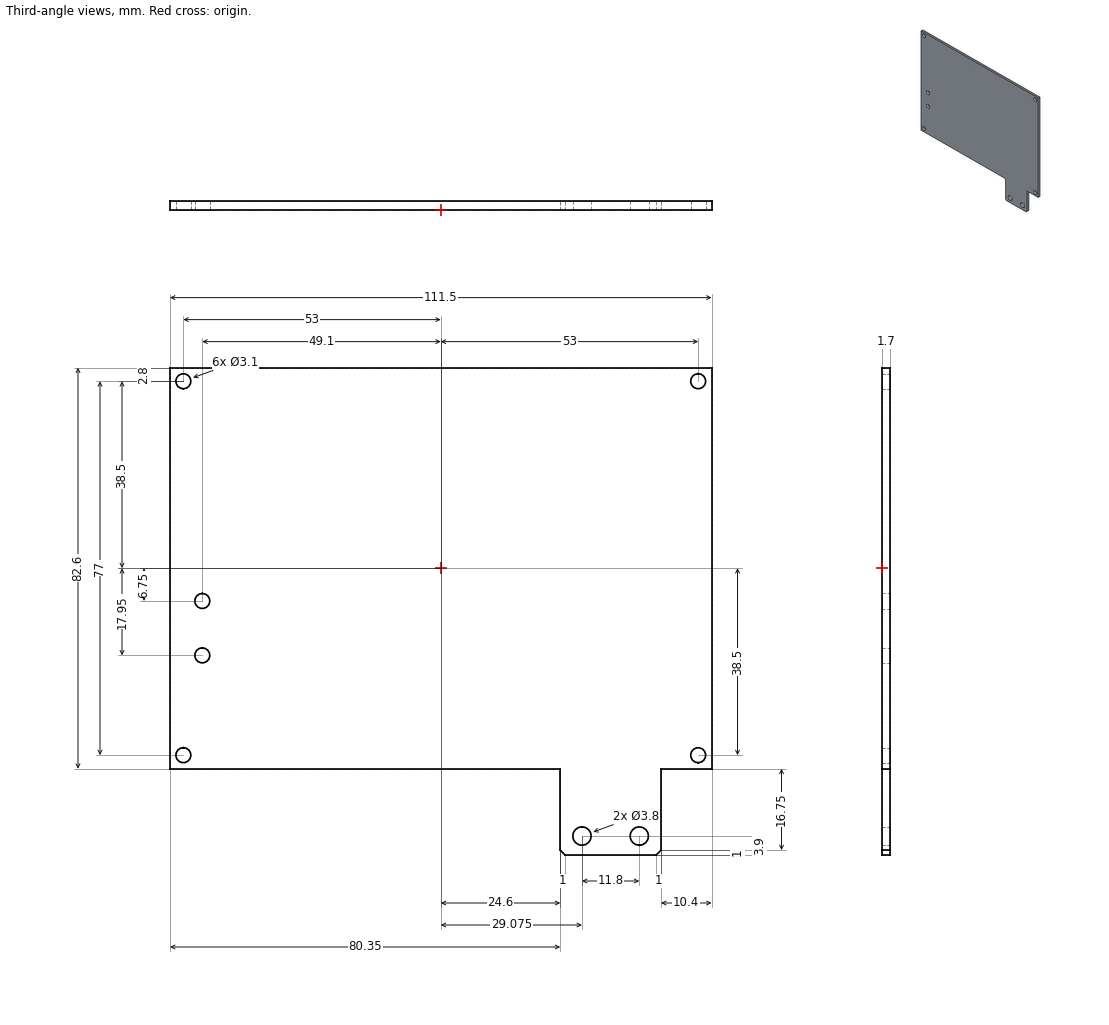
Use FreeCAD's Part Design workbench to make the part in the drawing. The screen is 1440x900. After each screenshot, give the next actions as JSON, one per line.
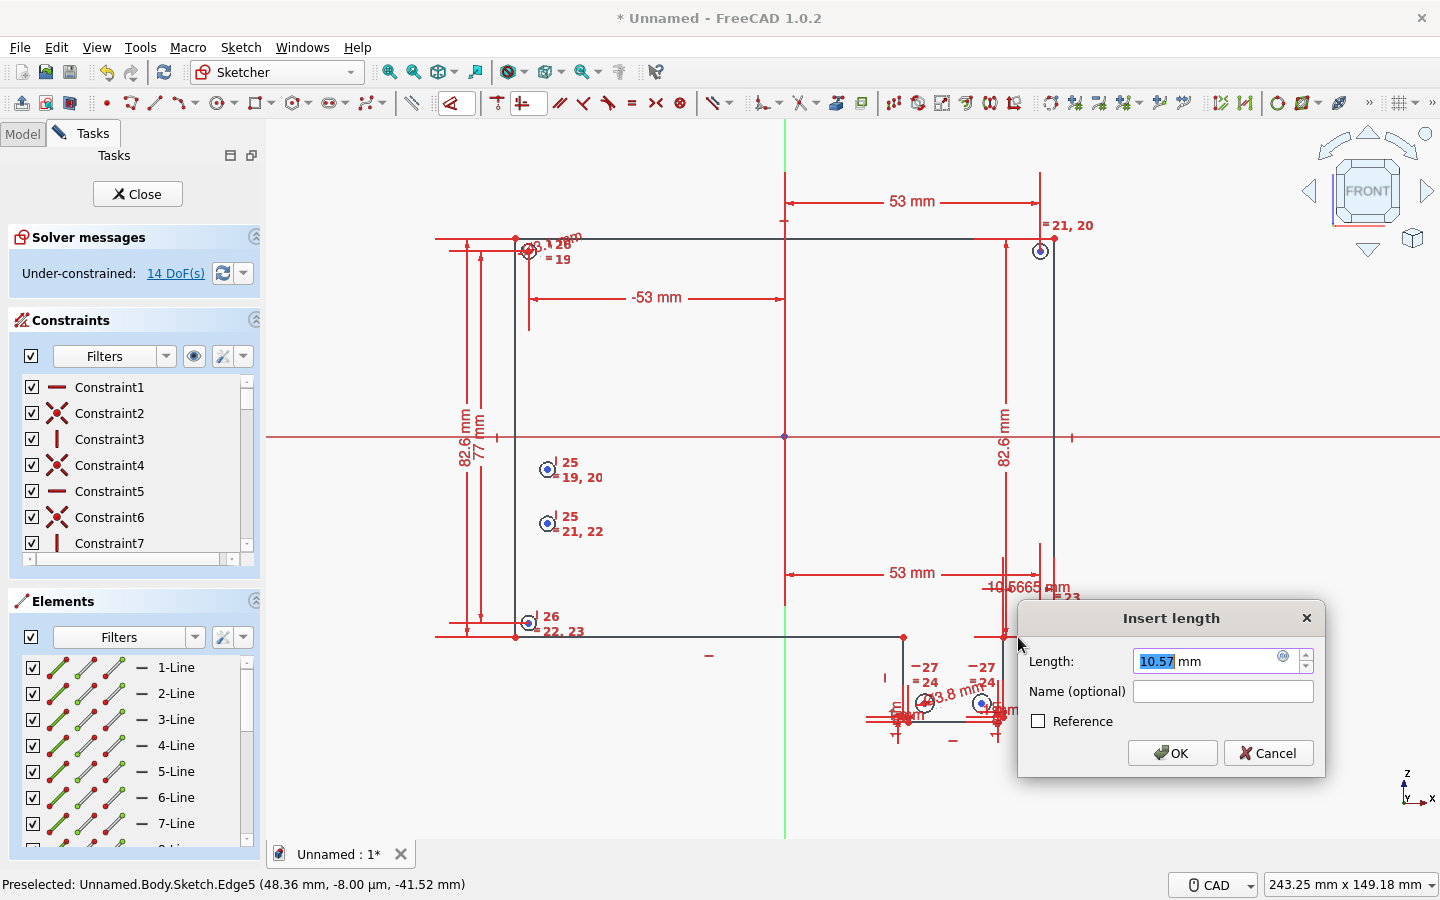
{"action": "type", "text": "10.4"}
{"action": "key", "text": "Return"}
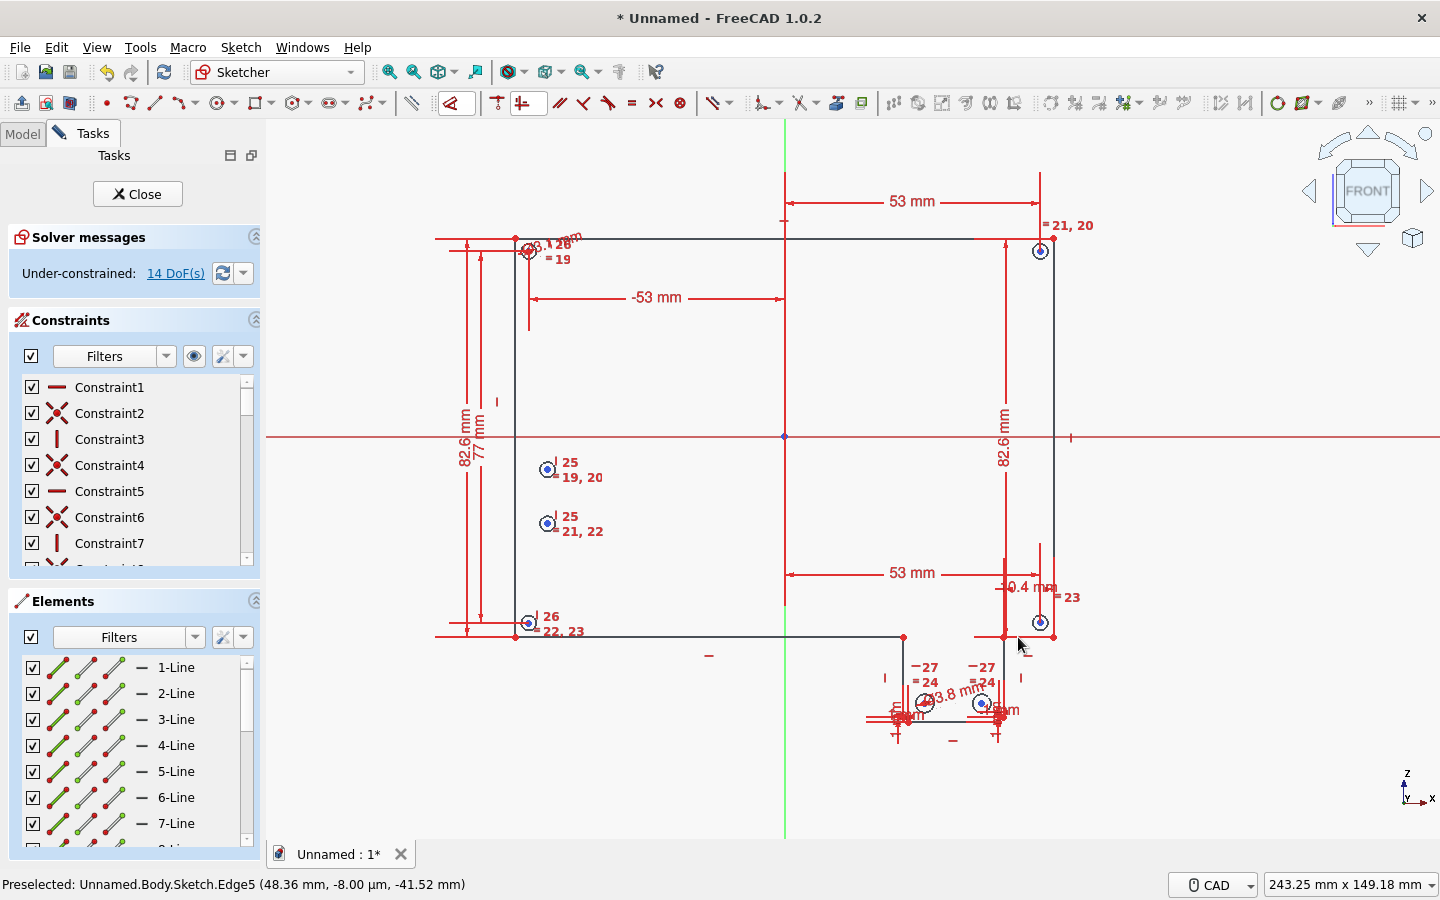
{"action": "left_click", "coordinate": [529, 251]}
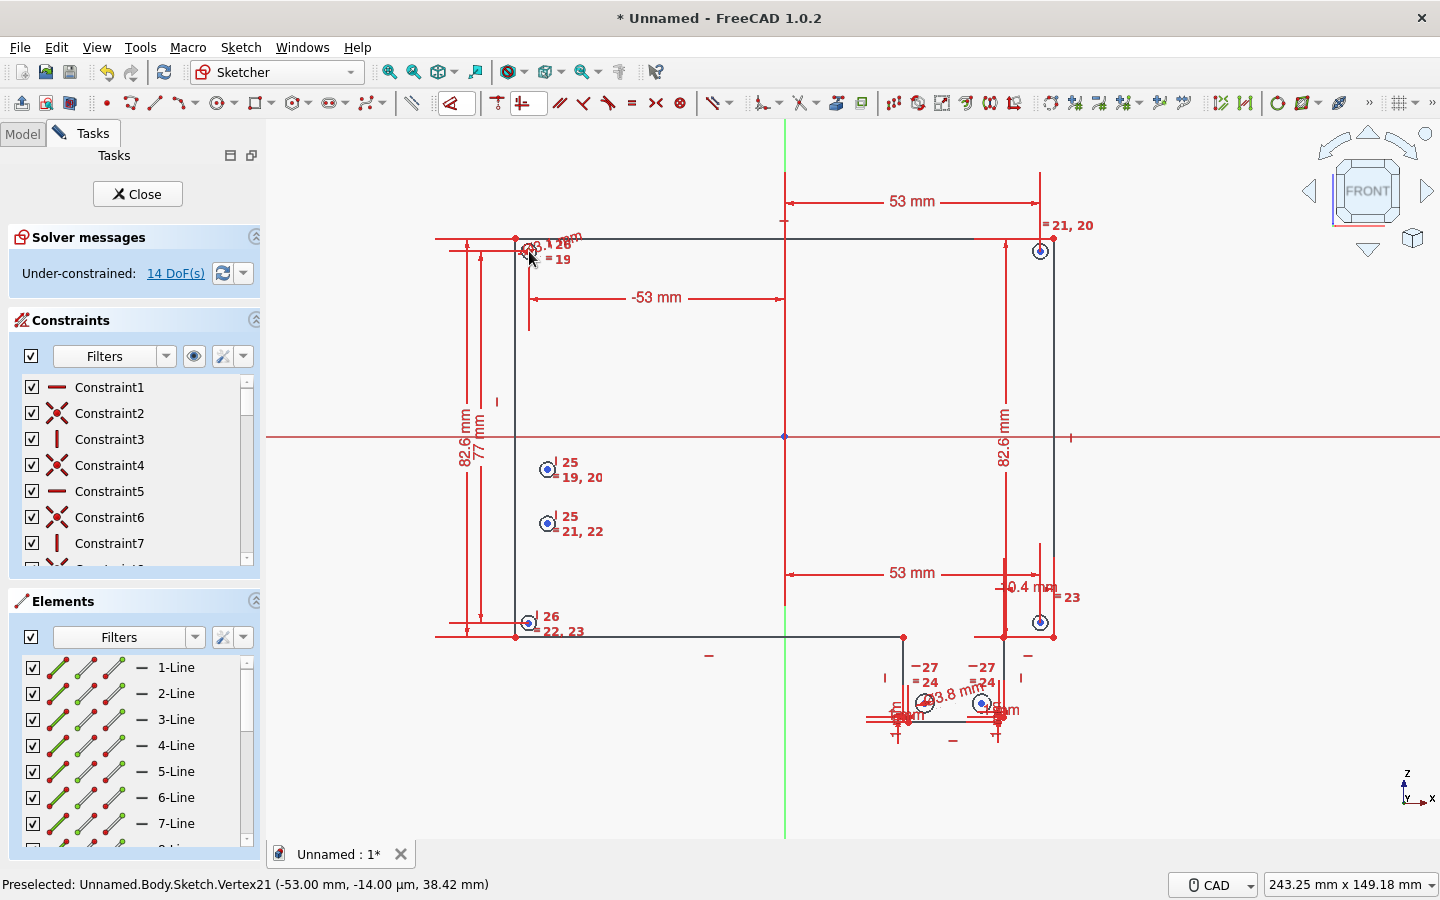
{"action": "key", "text": "i"}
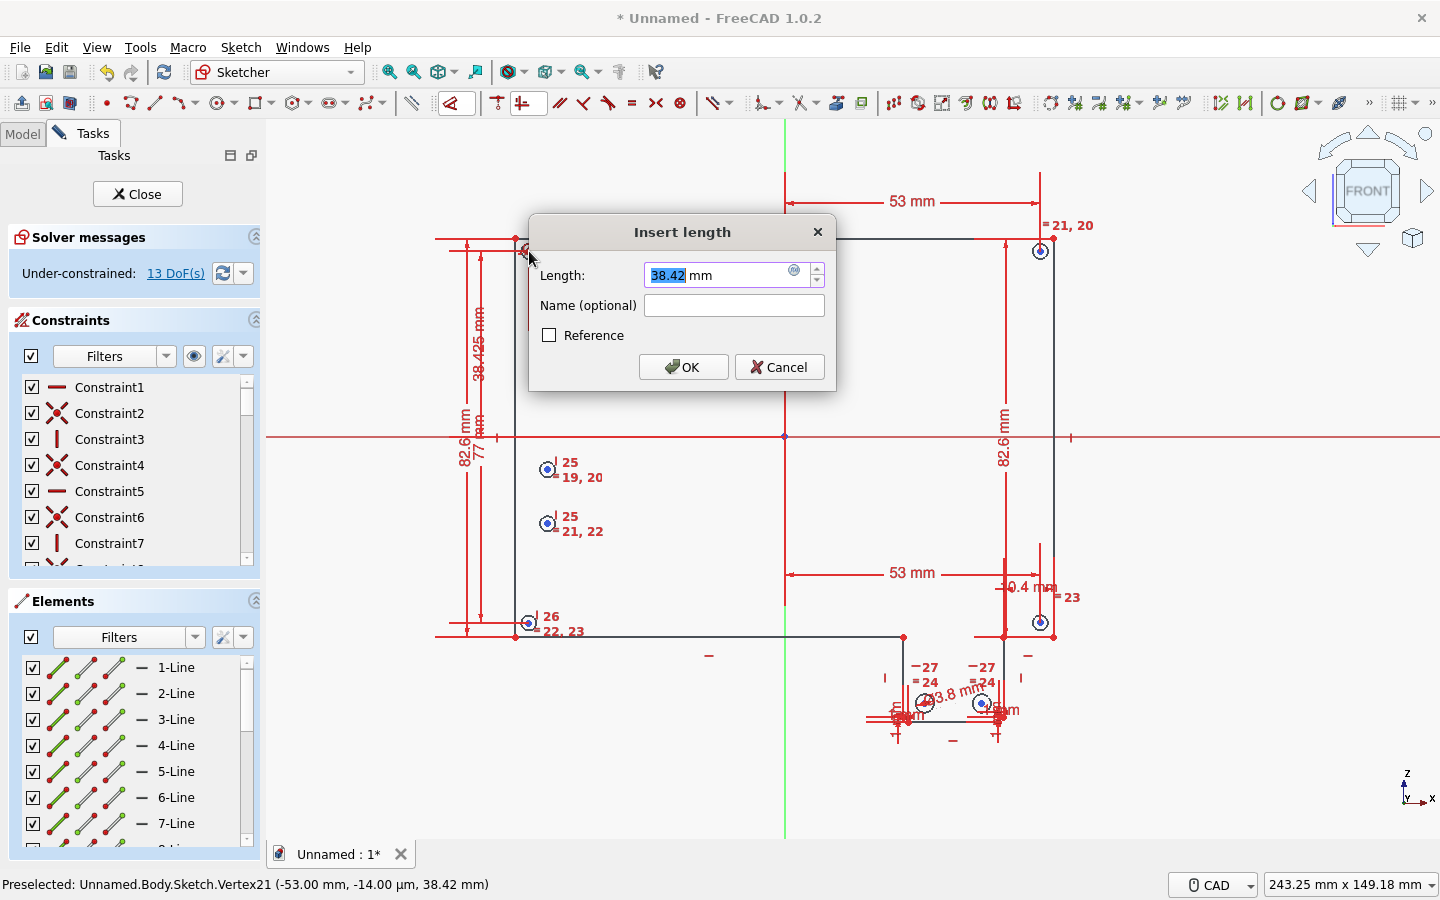
{"action": "type", "text": "38.5"}
{"action": "key", "text": "Return"}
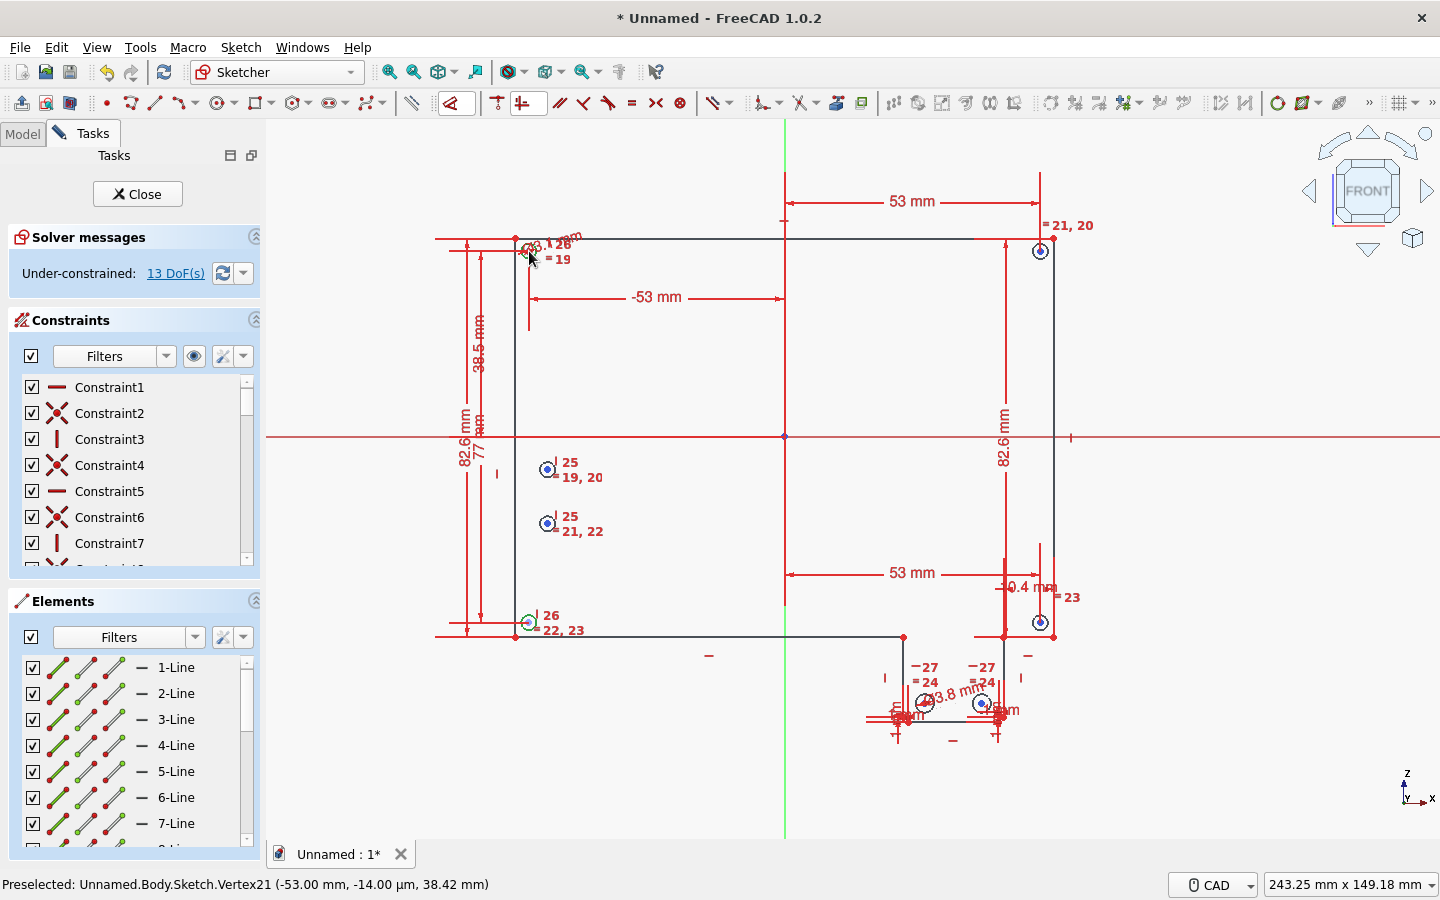
{"action": "left_click", "coordinate": [548, 470]}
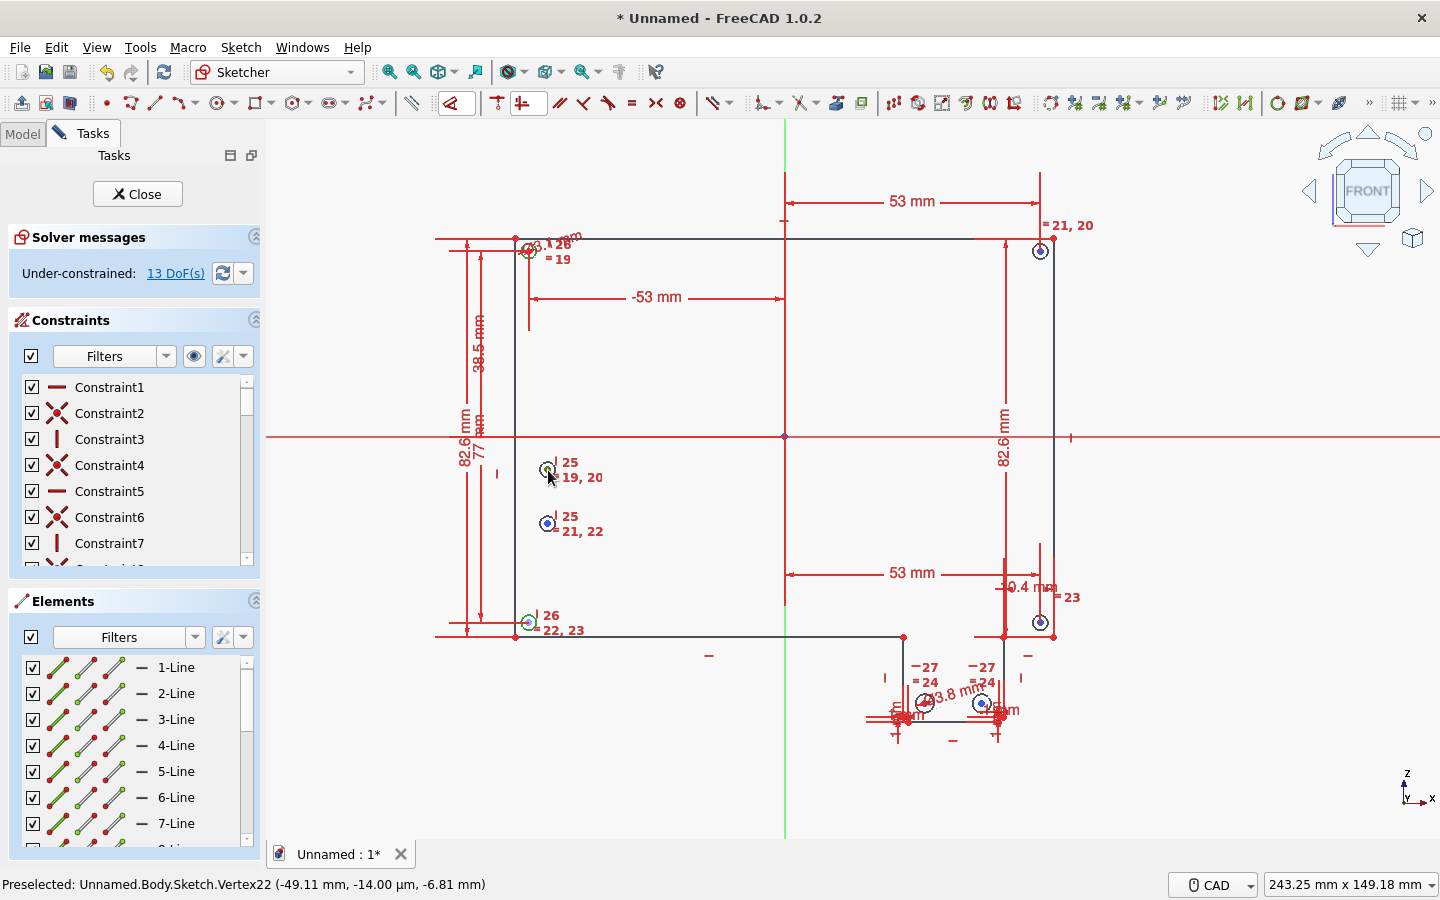
{"action": "left_click", "coordinate": [470, 104]}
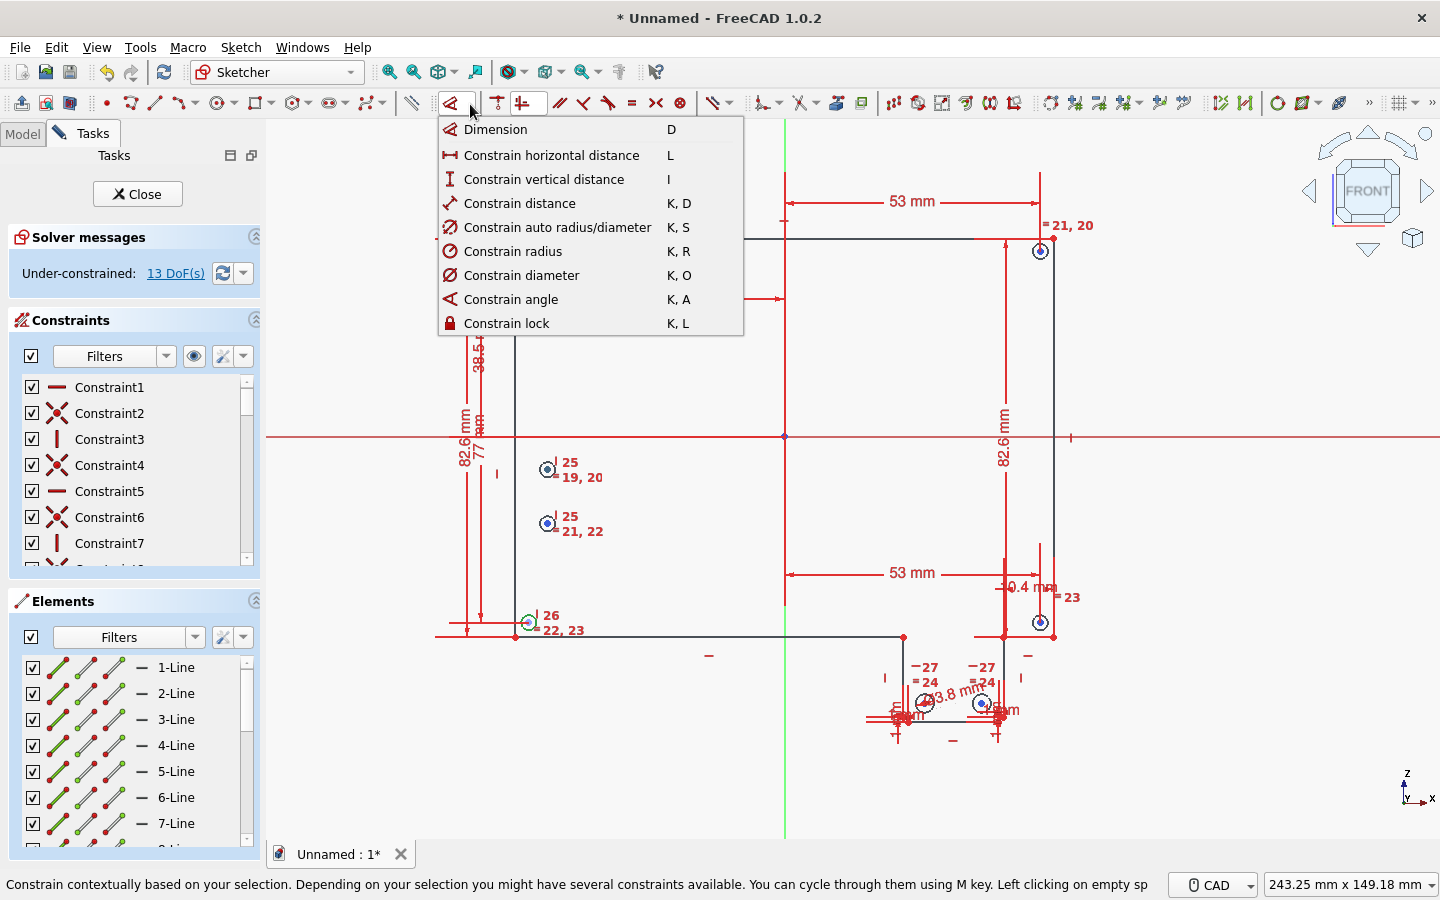
{"action": "left_click", "coordinate": [591, 155]}